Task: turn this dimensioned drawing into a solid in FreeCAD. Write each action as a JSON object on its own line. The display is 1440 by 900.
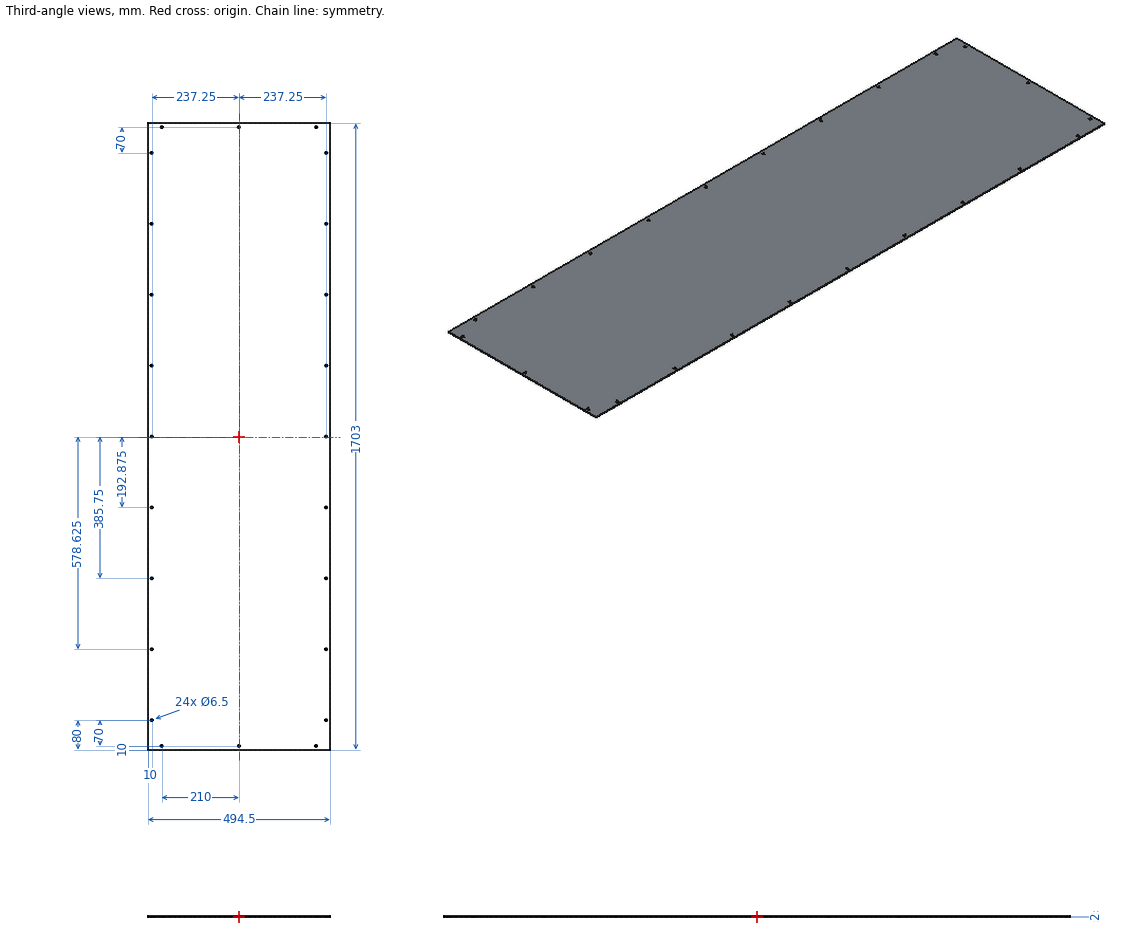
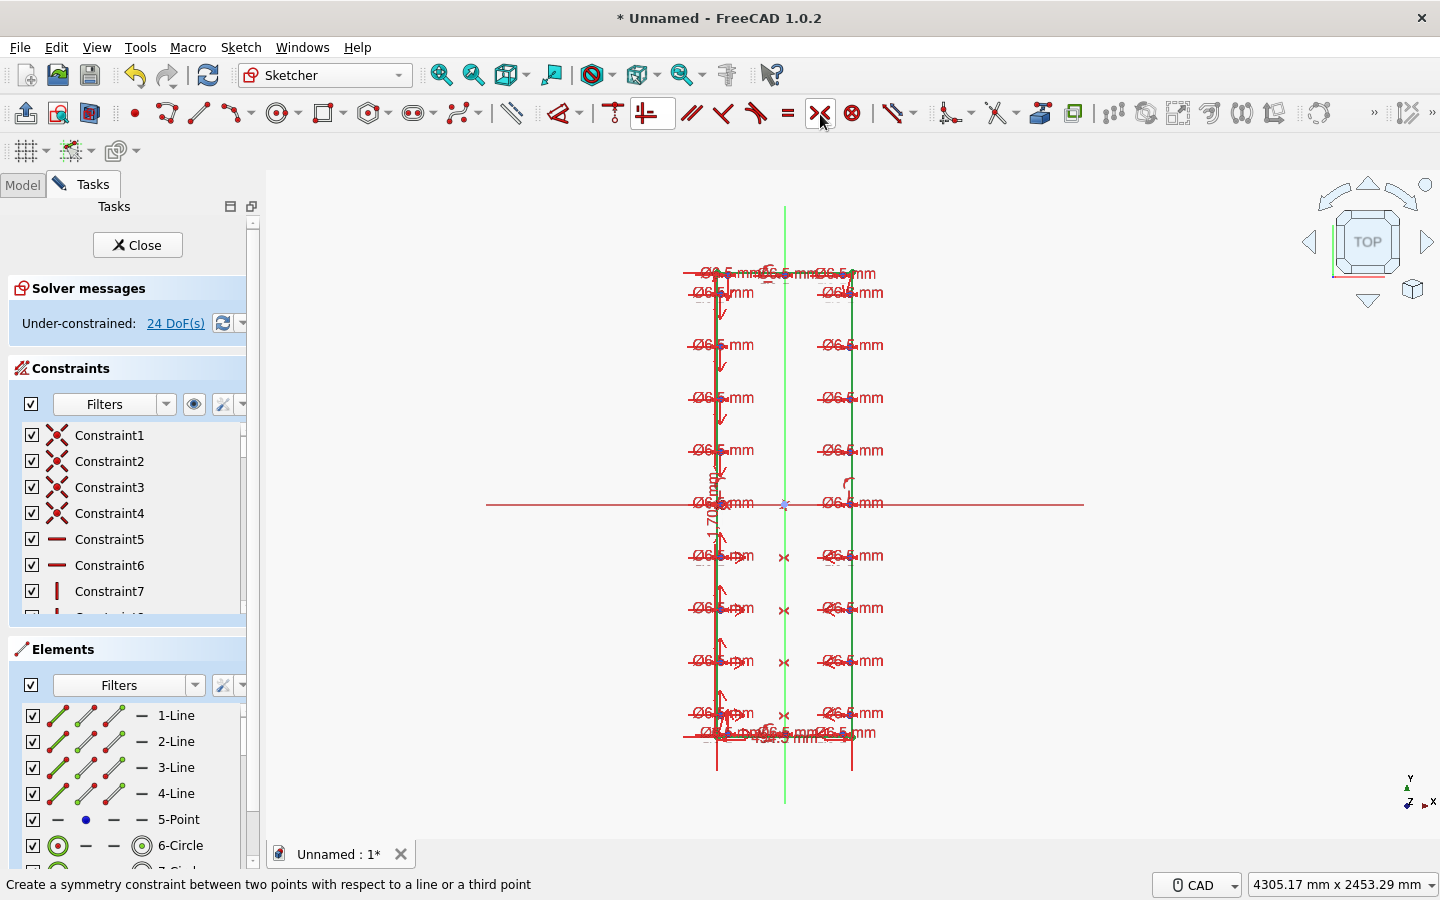
{"action": "left_click", "coordinate": [850, 558]}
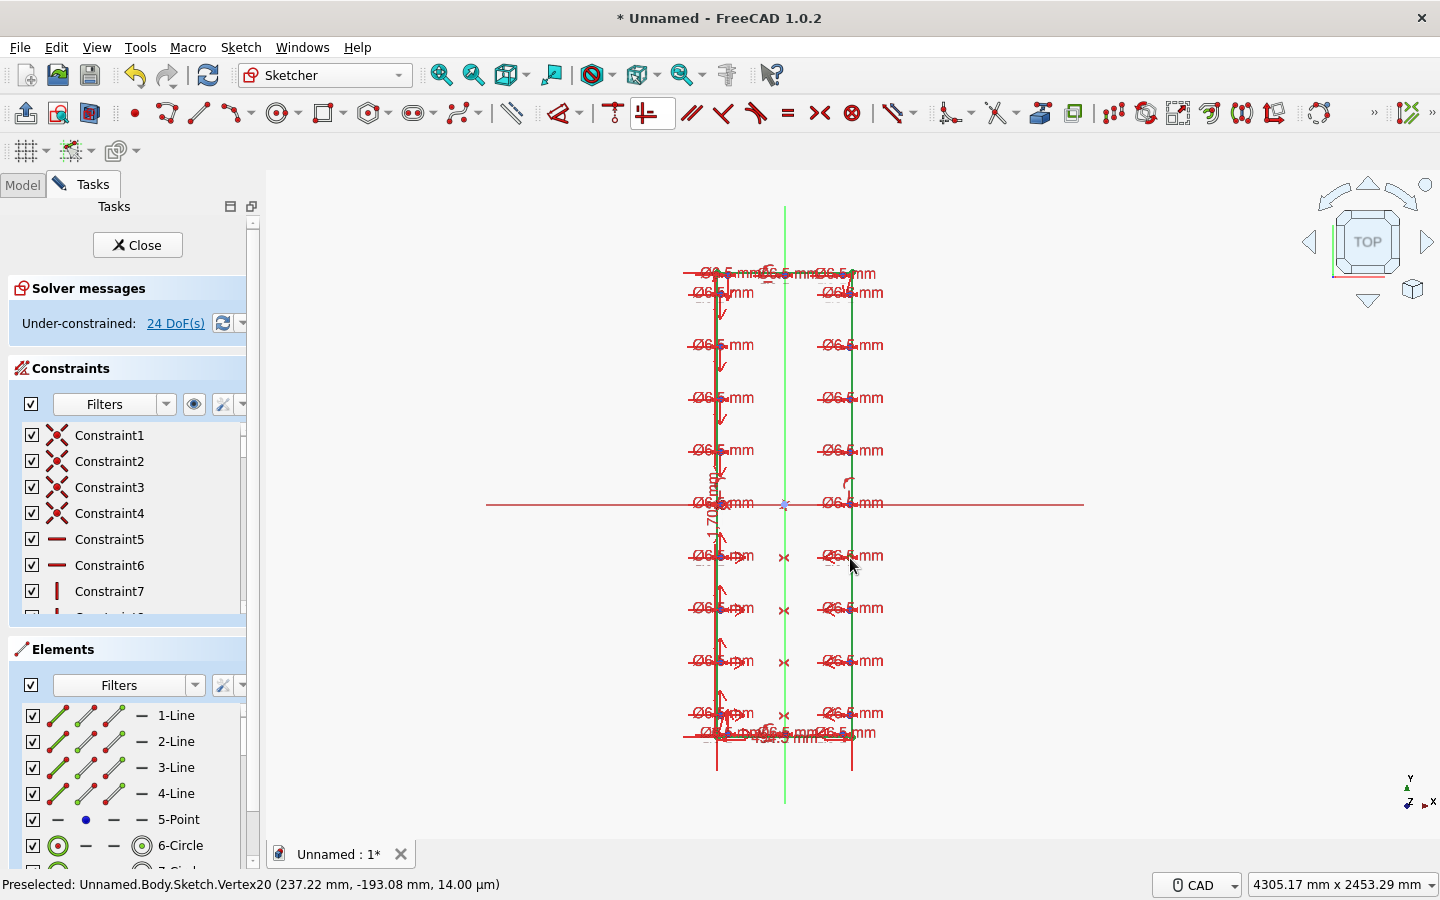
{"action": "left_click", "coordinate": [850, 452]}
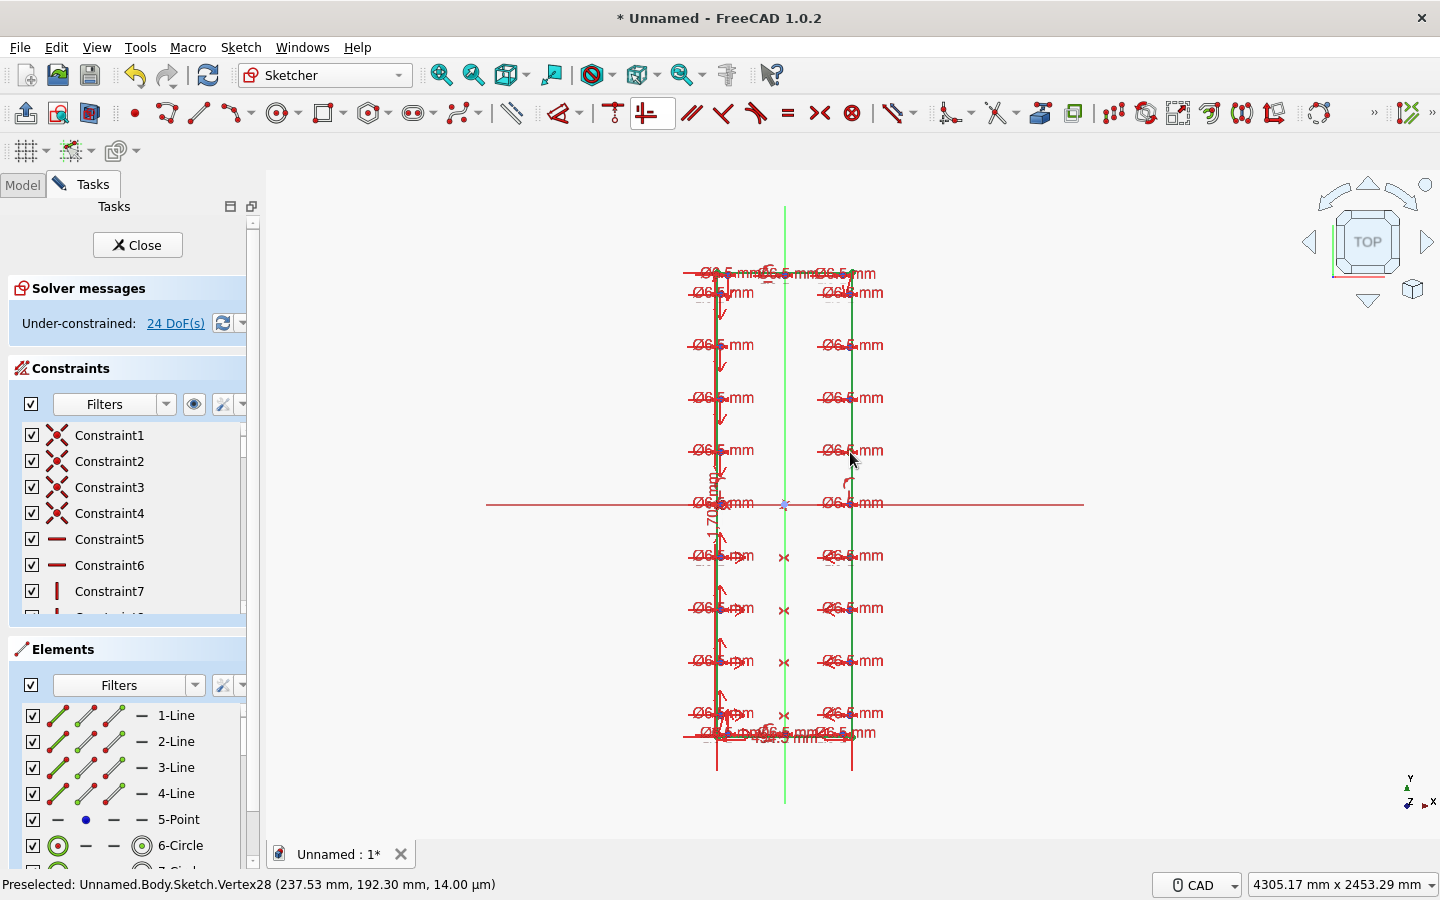
{"action": "left_click", "coordinate": [504, 505]}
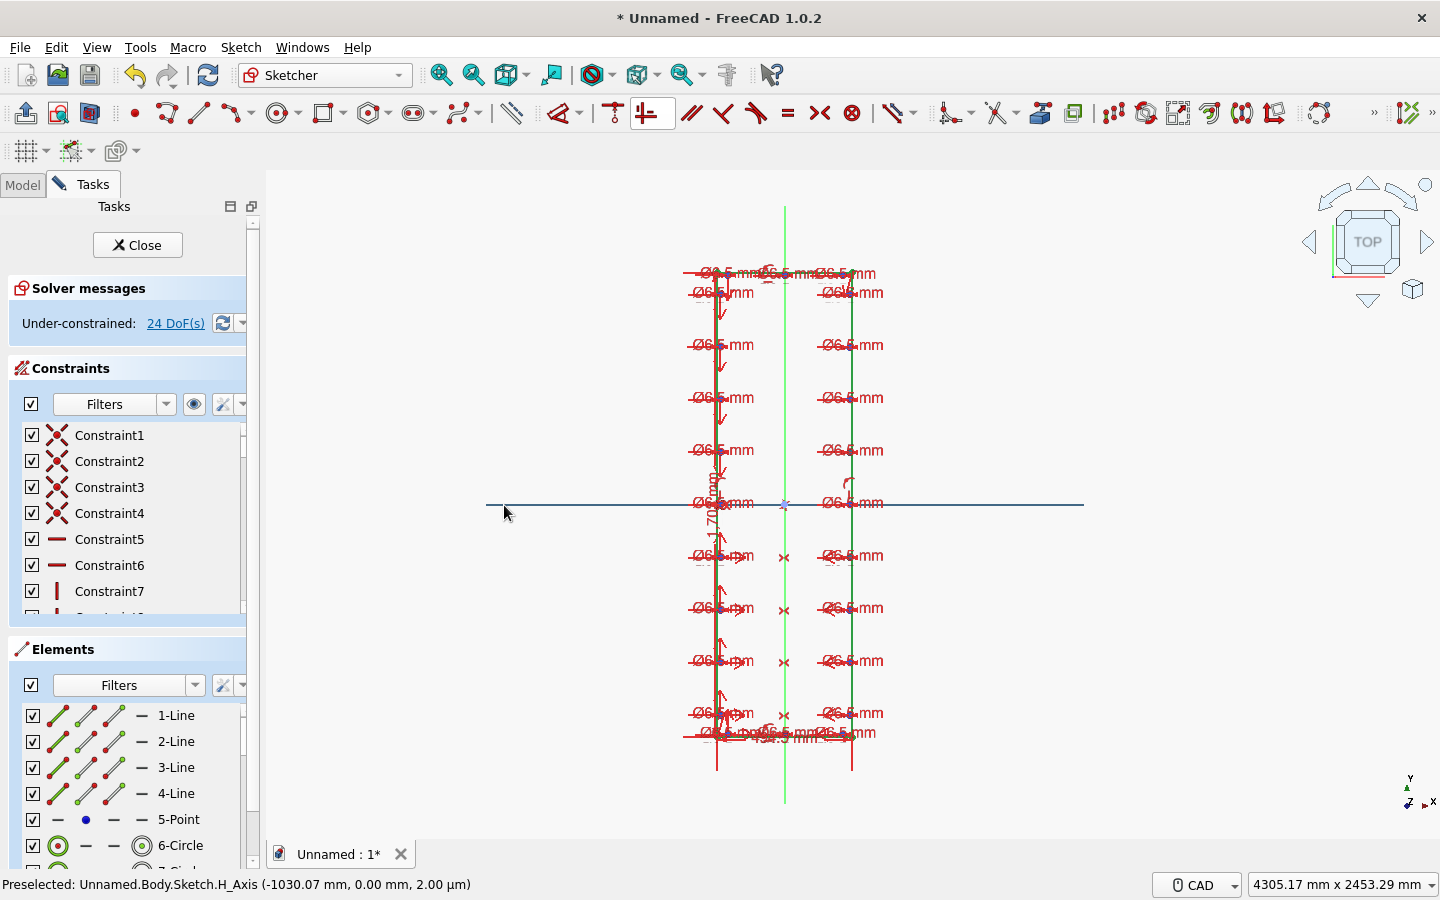
{"action": "left_click", "coordinate": [820, 114]}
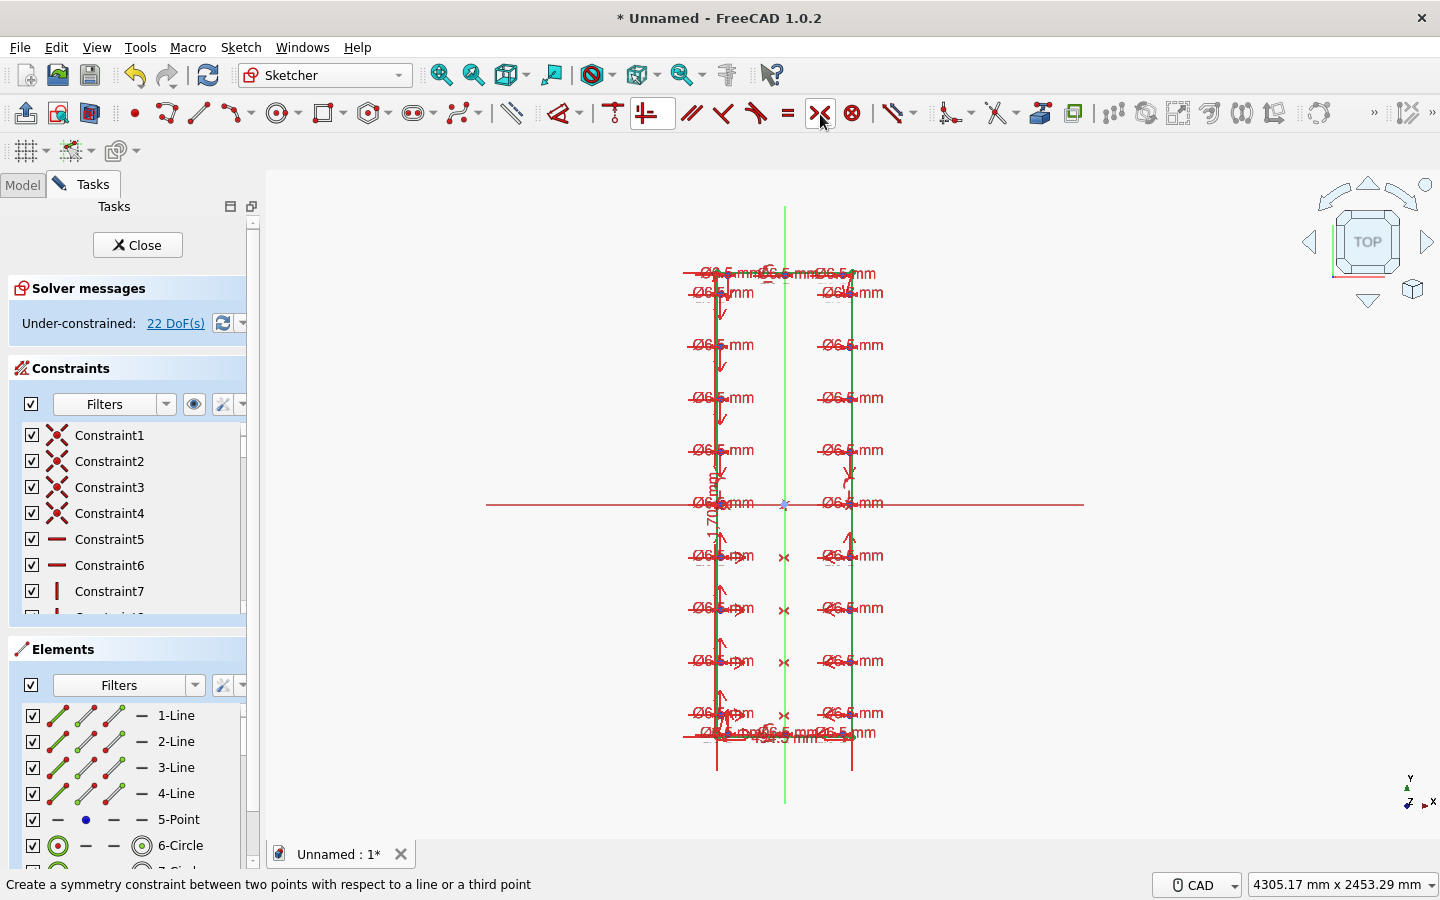
{"action": "left_click", "coordinate": [850, 610]}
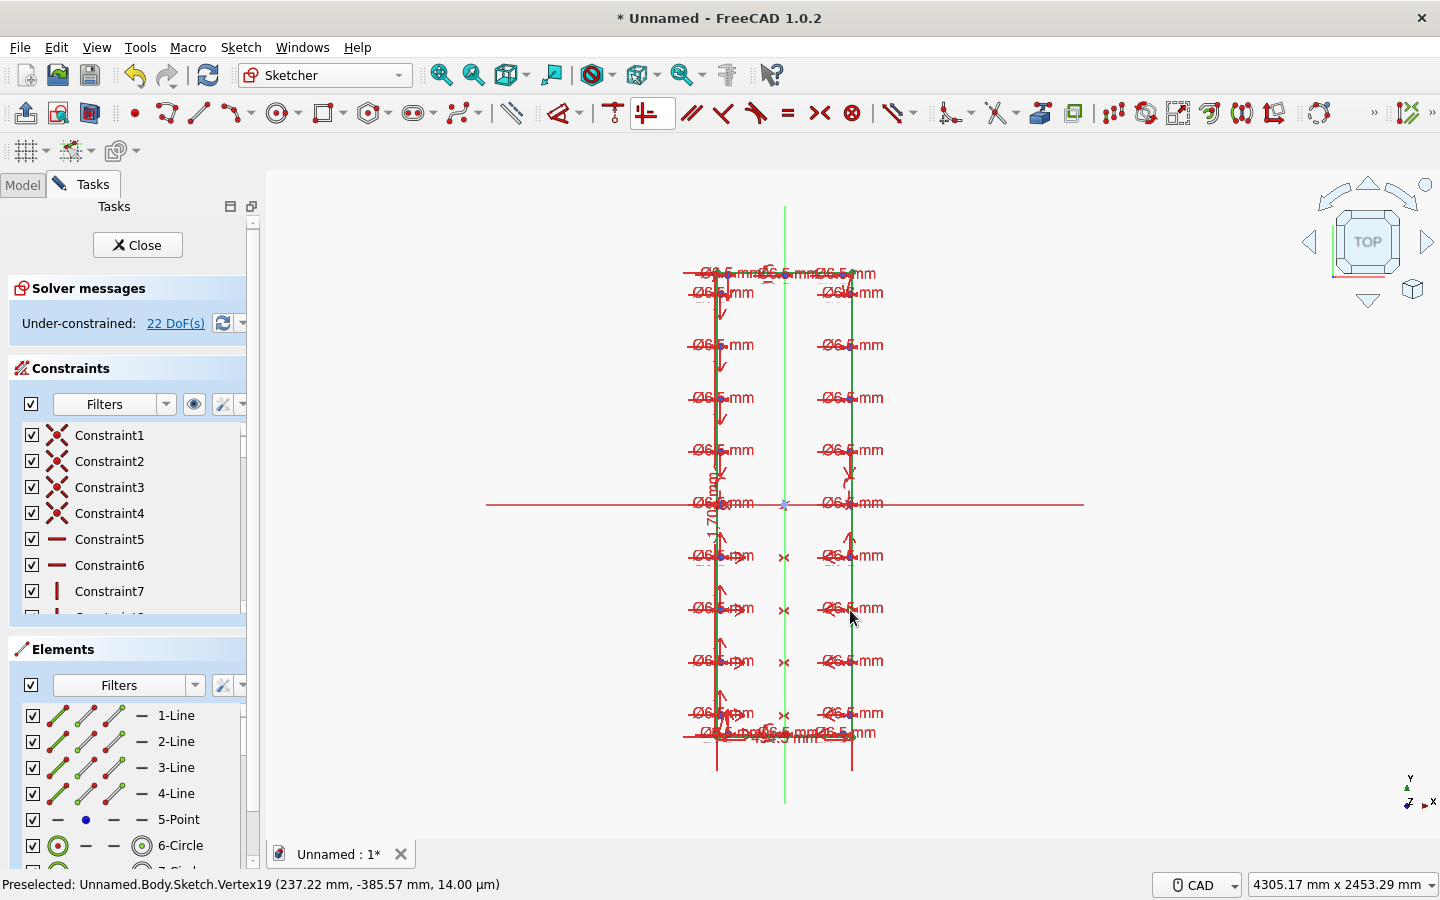
{"action": "left_click", "coordinate": [850, 400]}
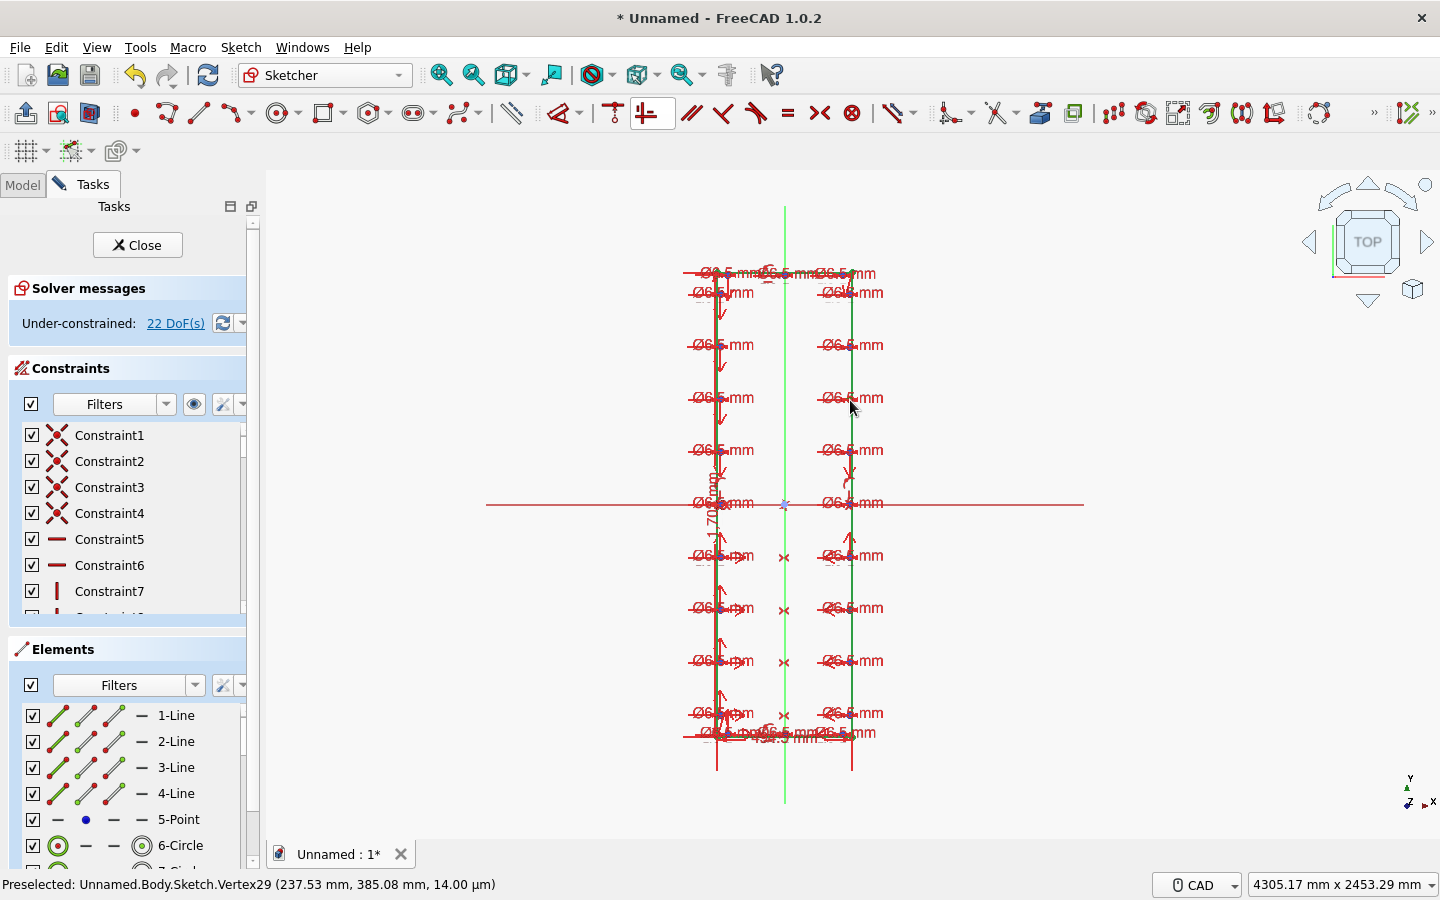
{"action": "left_click", "coordinate": [504, 505]}